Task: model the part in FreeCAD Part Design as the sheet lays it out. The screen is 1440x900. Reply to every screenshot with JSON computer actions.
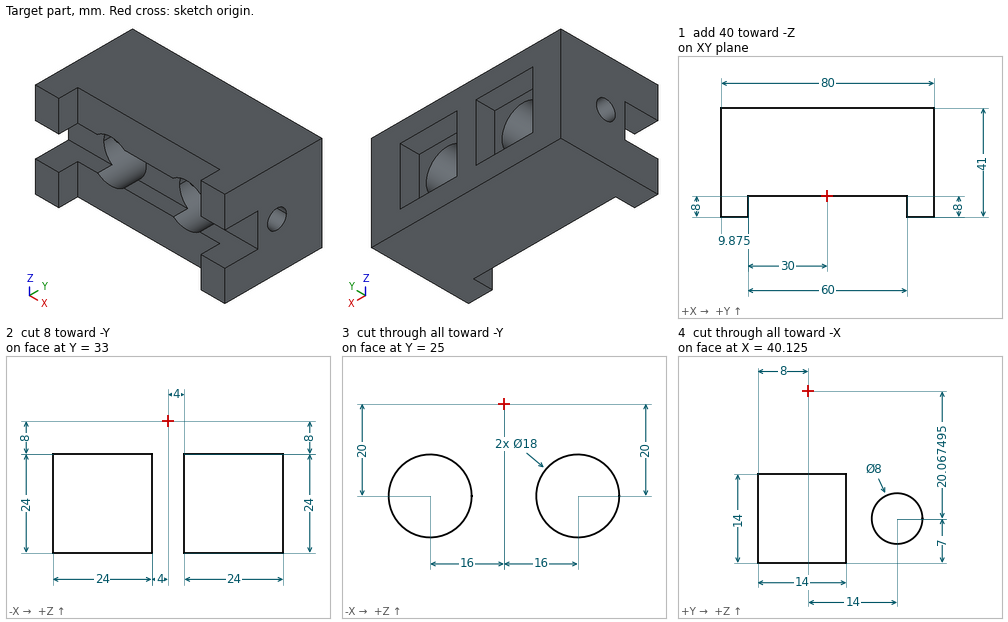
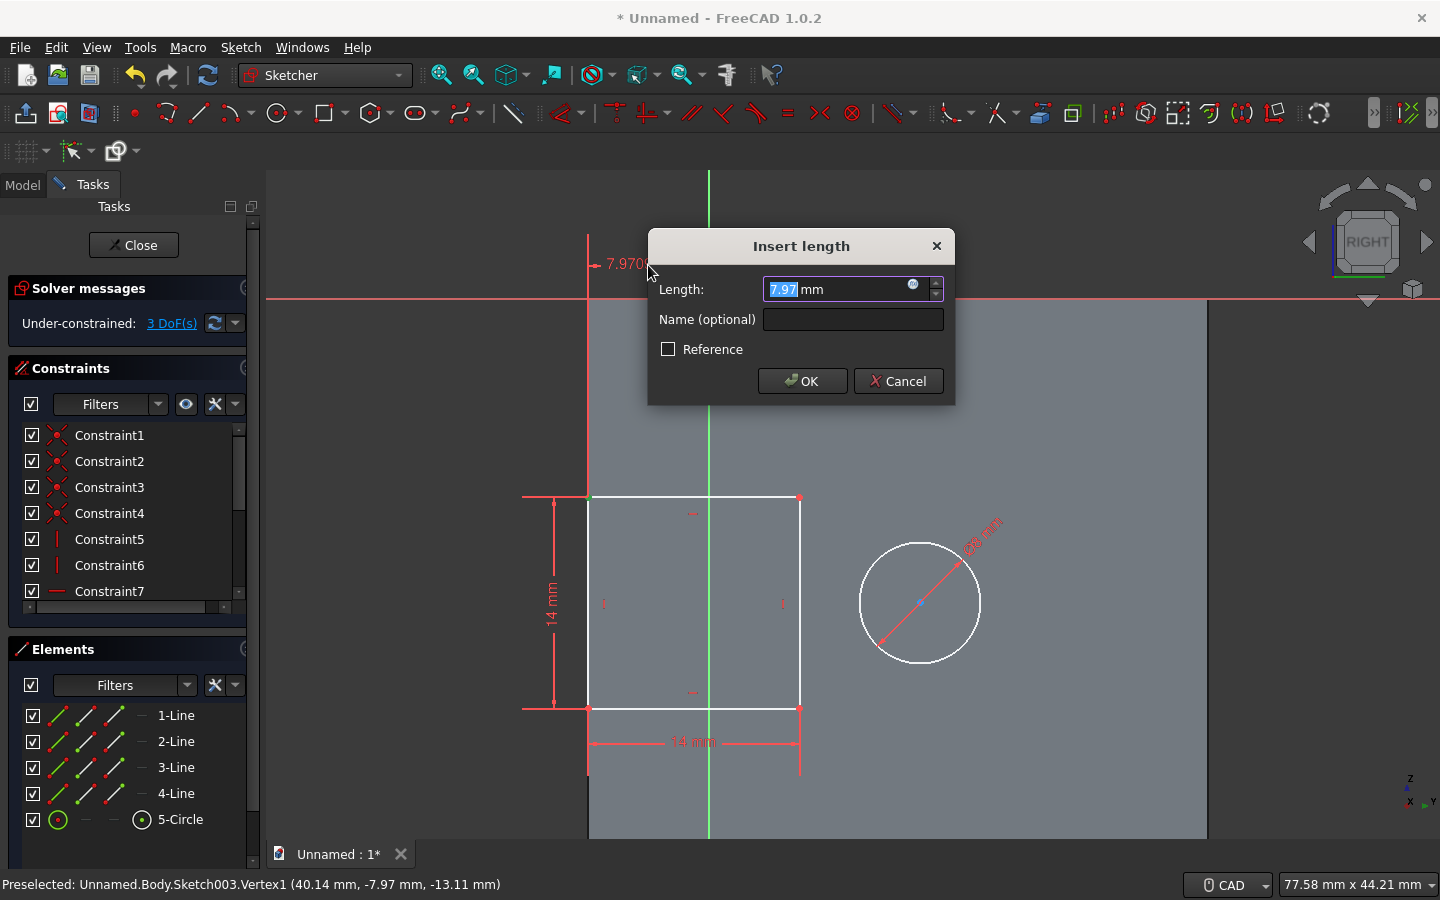
{"action": "type", "text": "8"}
{"action": "key", "text": "Return"}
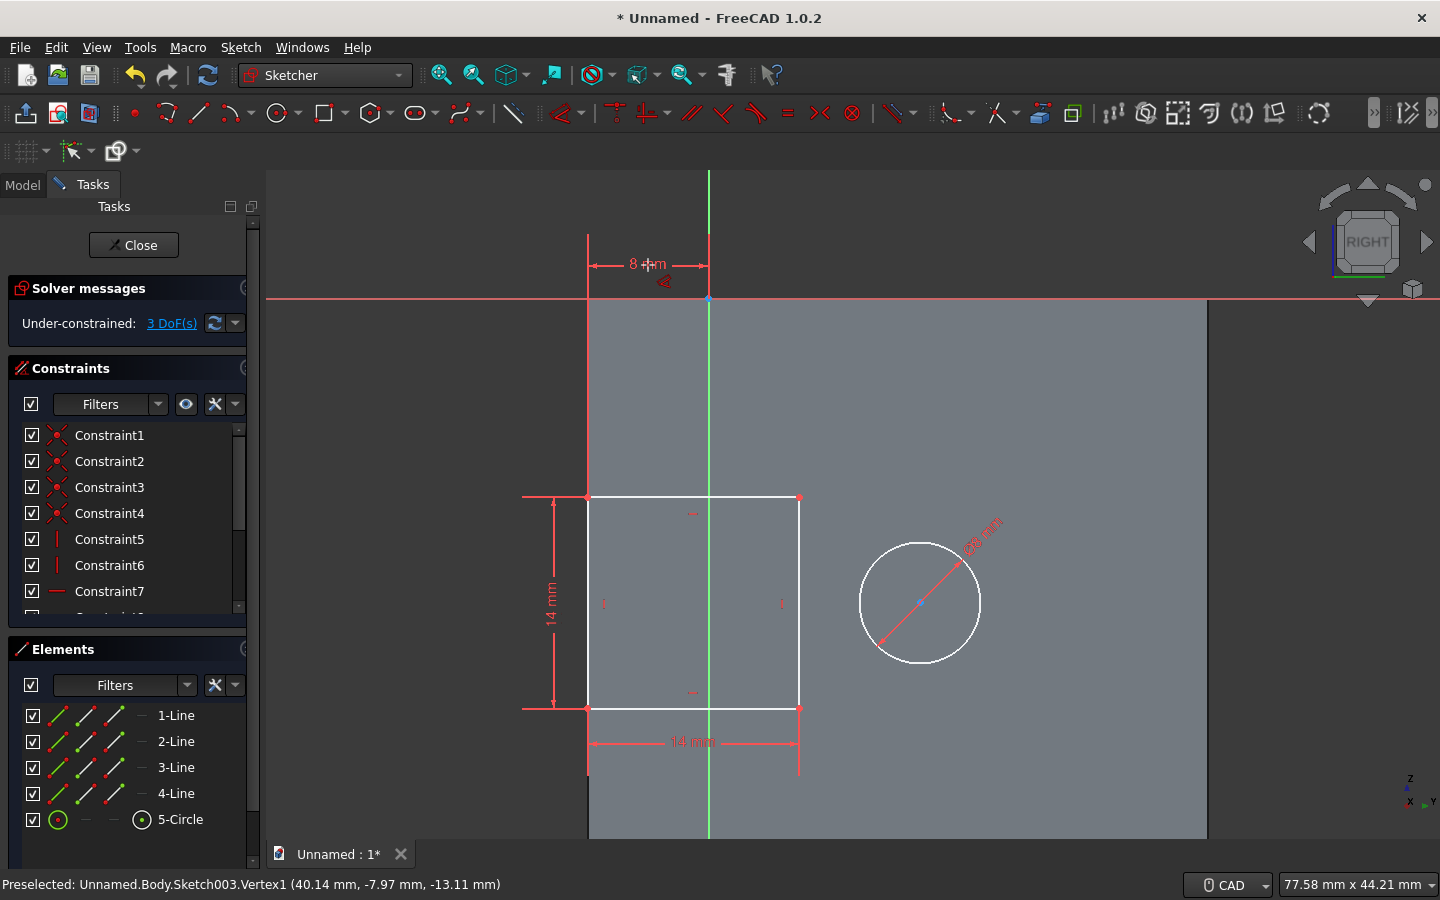
{"action": "left_click", "coordinate": [920, 603]}
{"action": "left_click", "coordinate": [814, 265]}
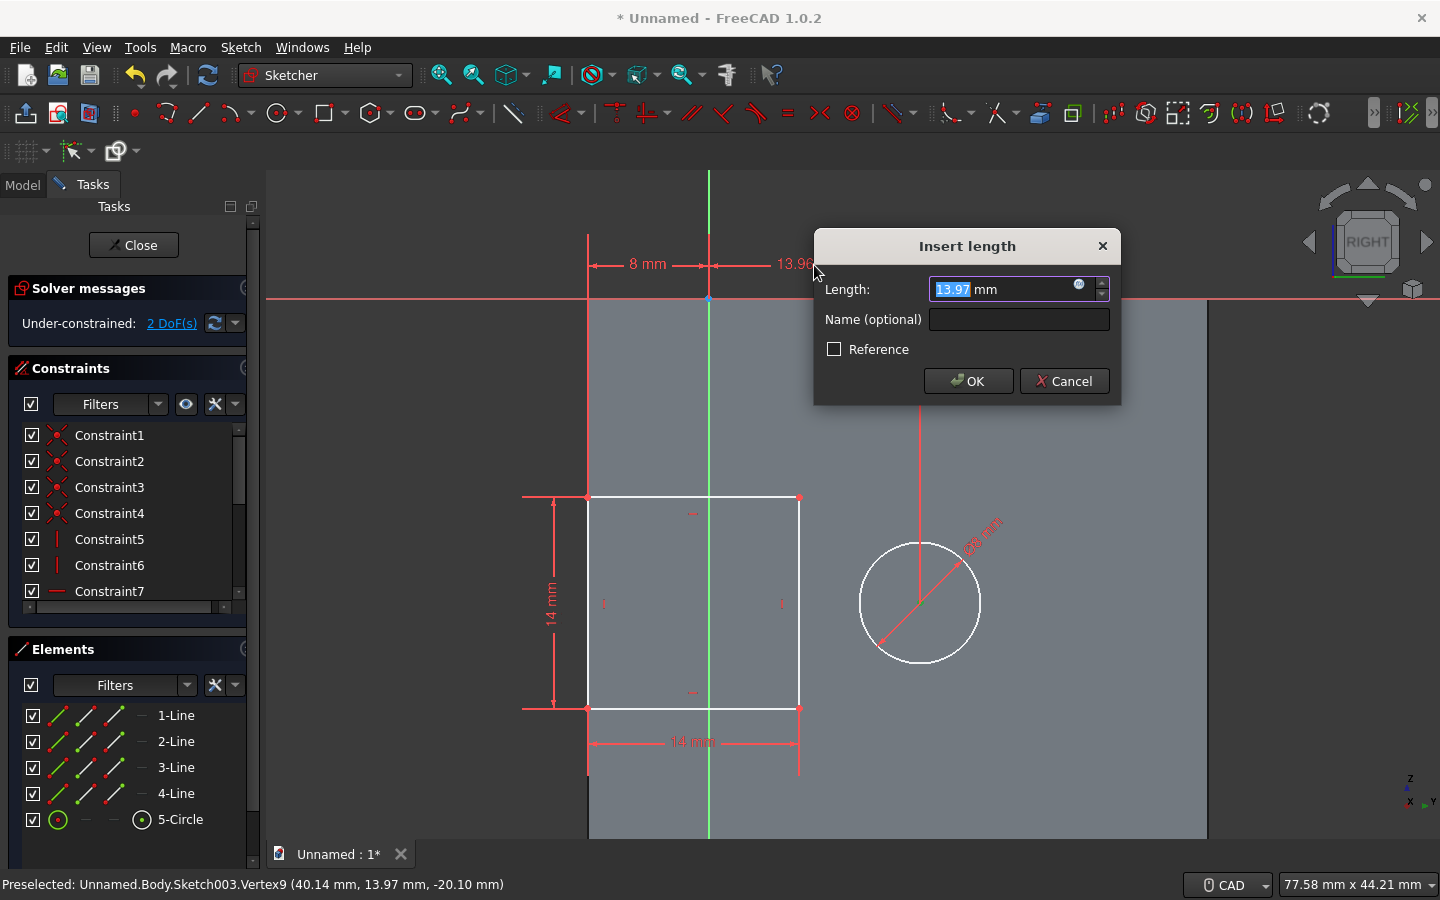
{"action": "type", "text": "14"}
{"action": "key", "text": "Return"}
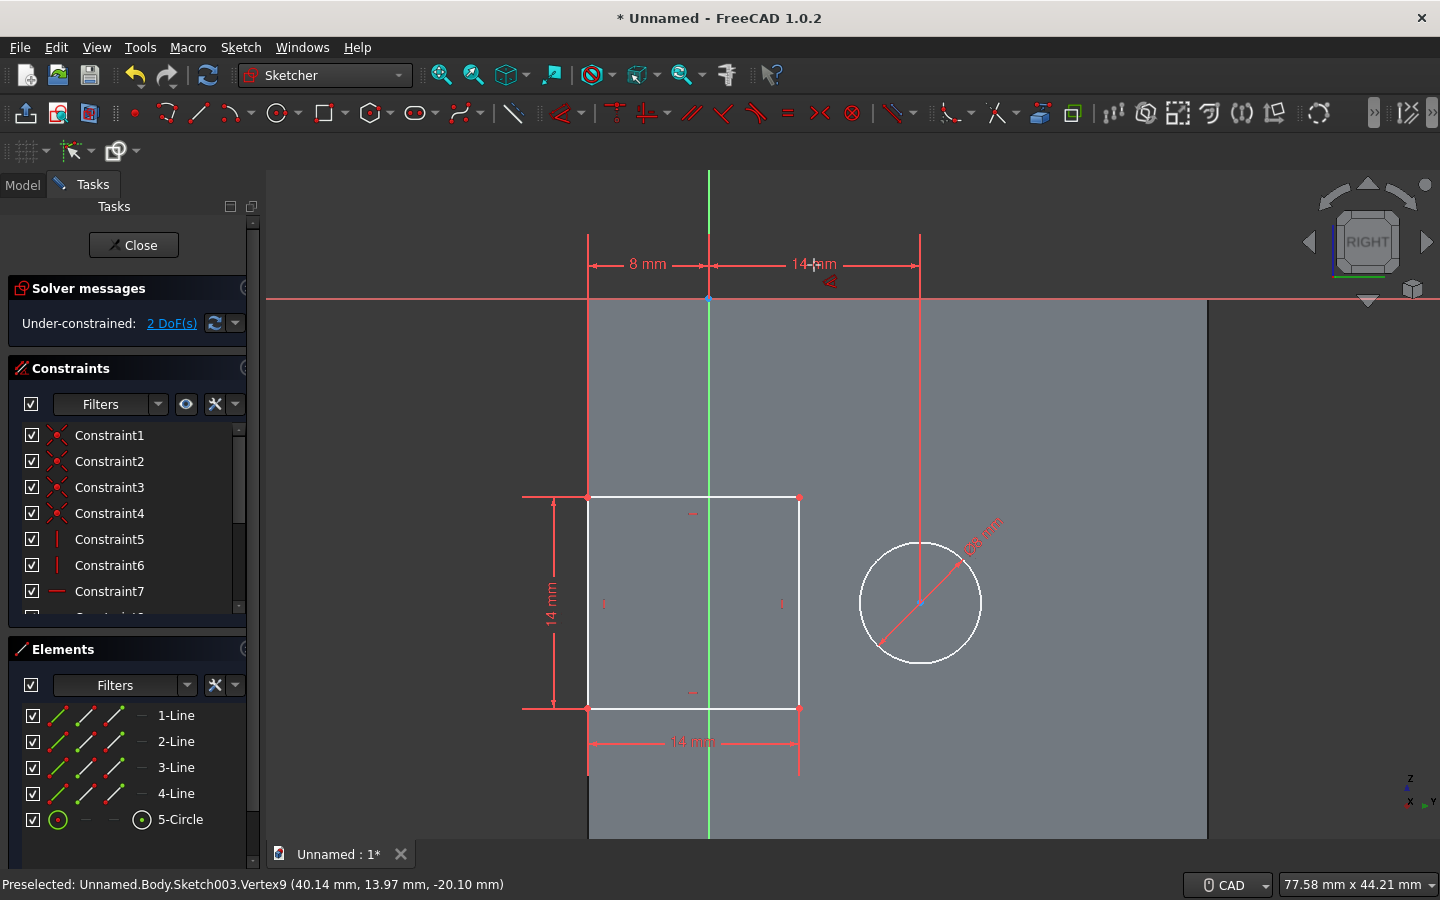
{"action": "left_click", "coordinate": [799, 709]}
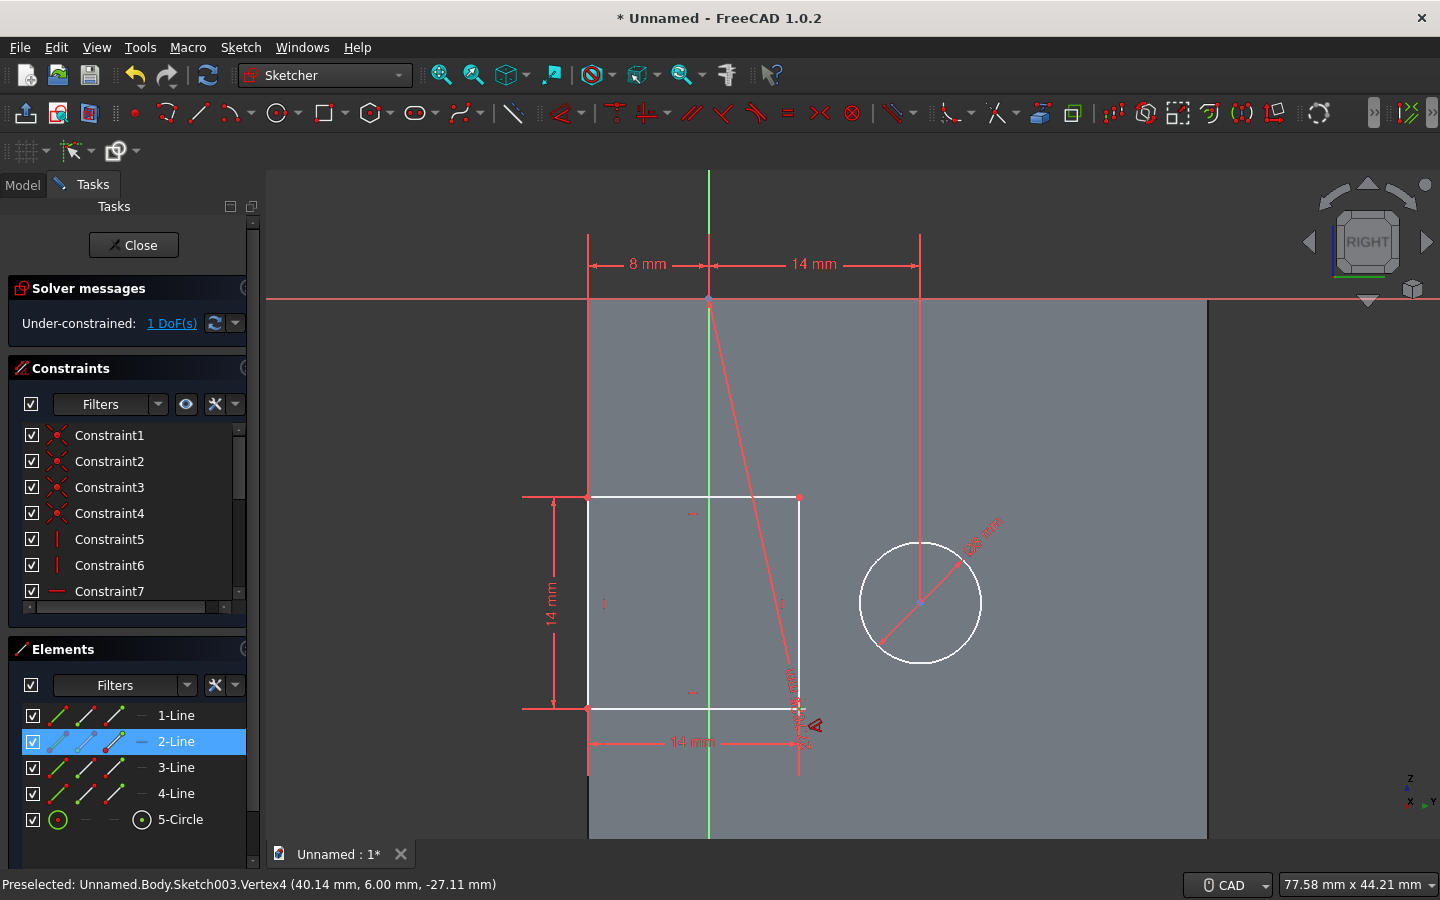
{"action": "left_click", "coordinate": [920, 603]}
{"action": "left_click", "coordinate": [954, 632]}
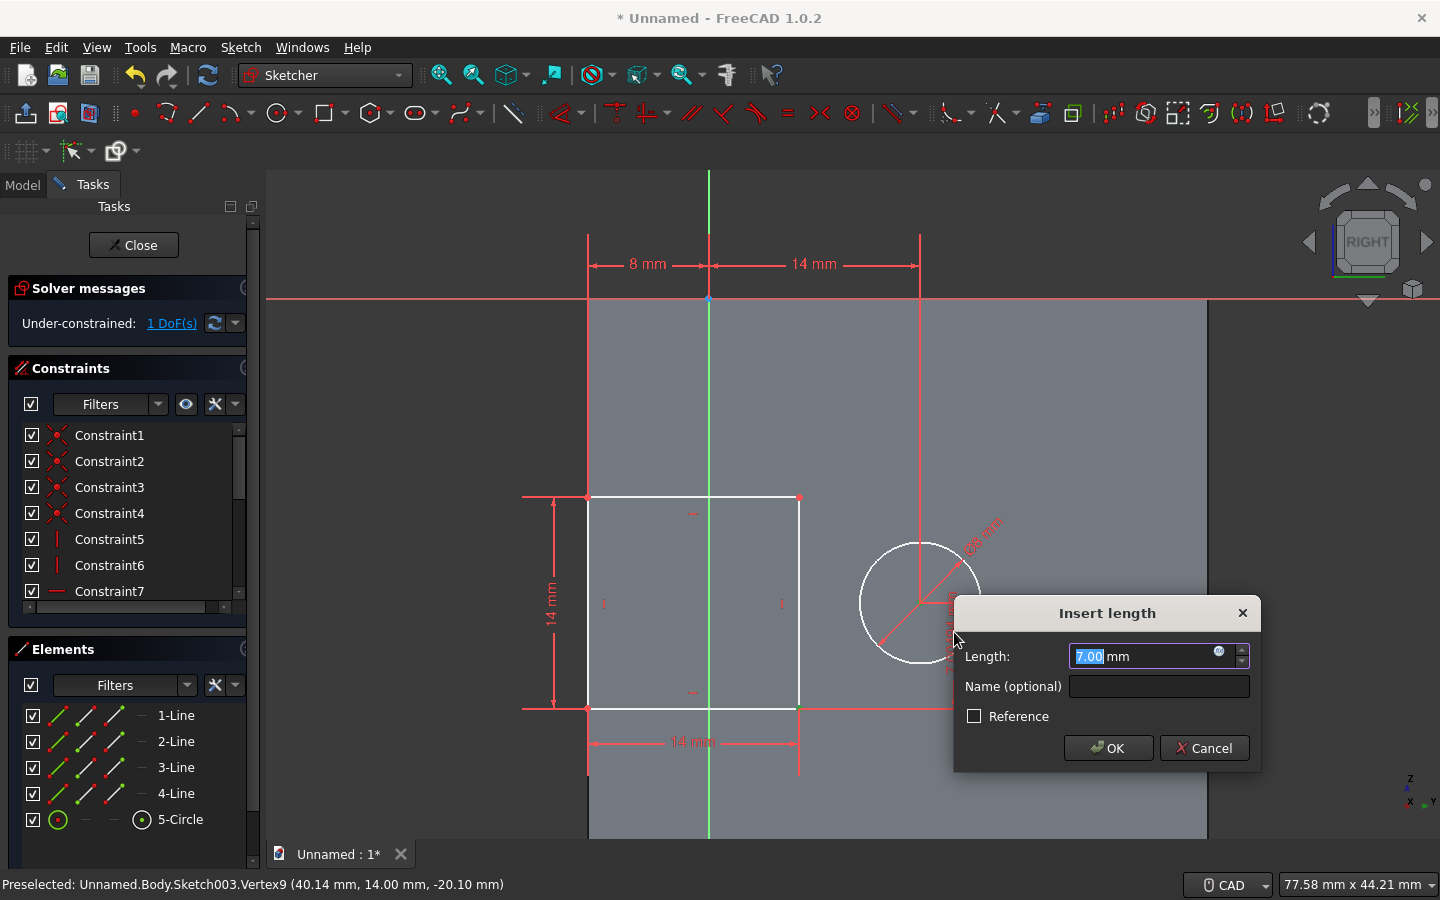
{"action": "type", "text": "7"}
{"action": "key", "text": "Return"}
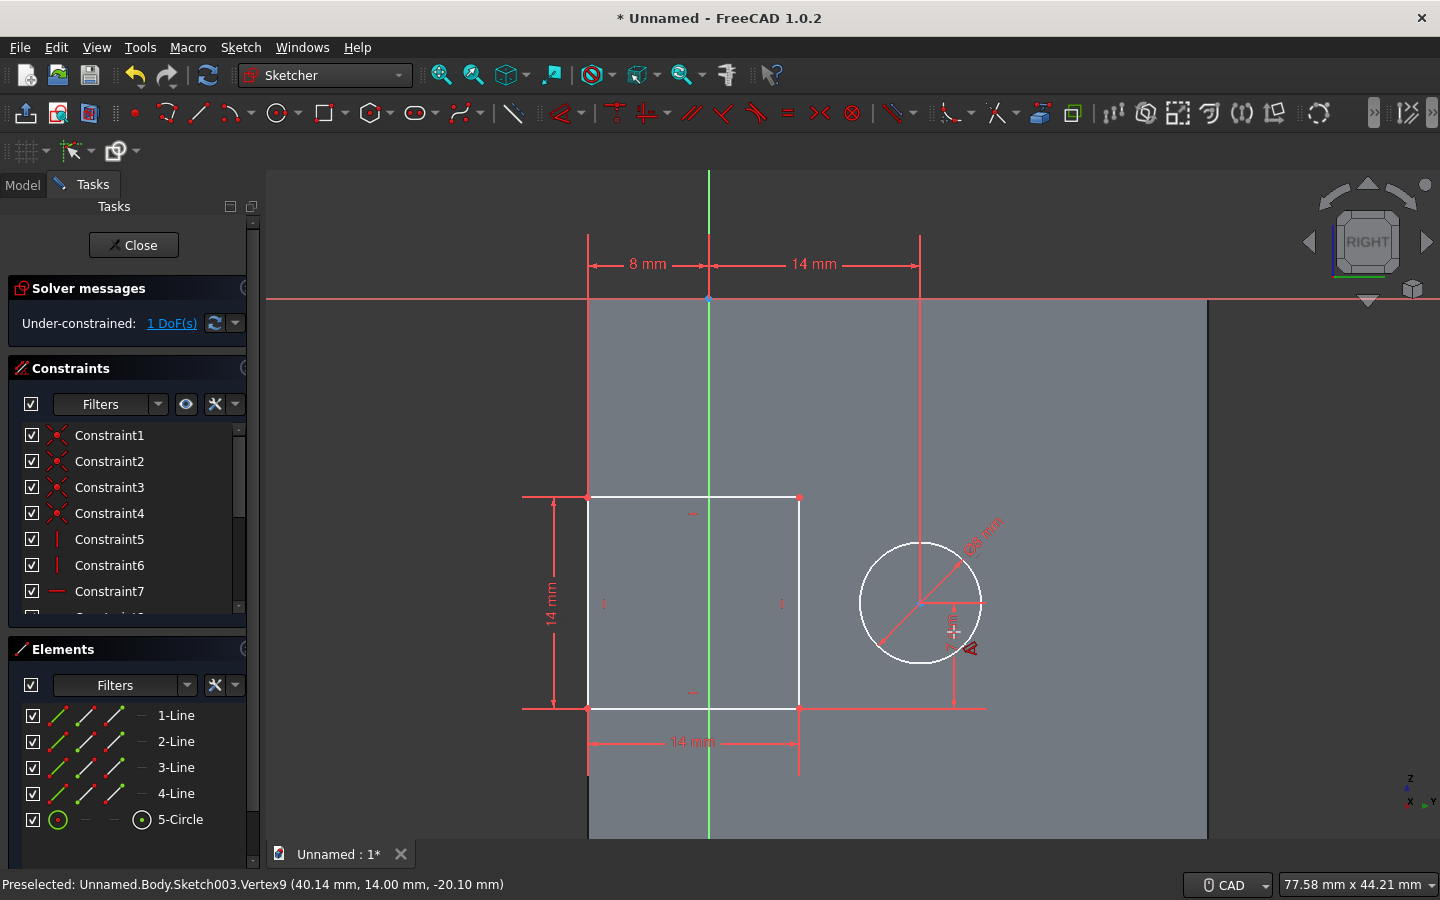
{"action": "left_click", "coordinate": [920, 603]}
{"action": "left_click", "coordinate": [954, 451]}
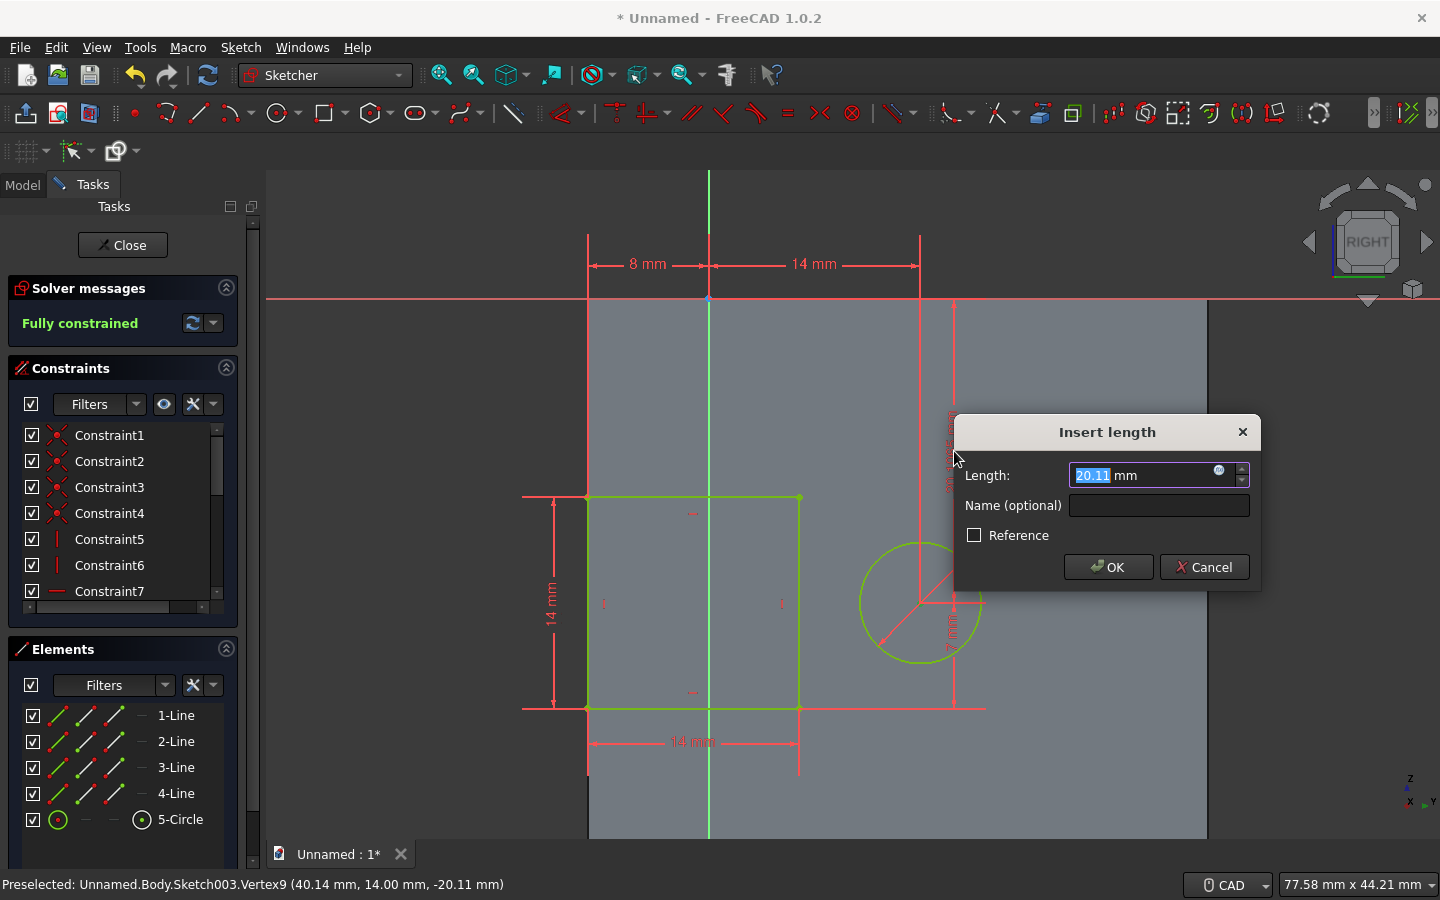
{"action": "type", "text": "20.067495"}
{"action": "key", "text": "Return"}
{"action": "key", "text": "Escape"}